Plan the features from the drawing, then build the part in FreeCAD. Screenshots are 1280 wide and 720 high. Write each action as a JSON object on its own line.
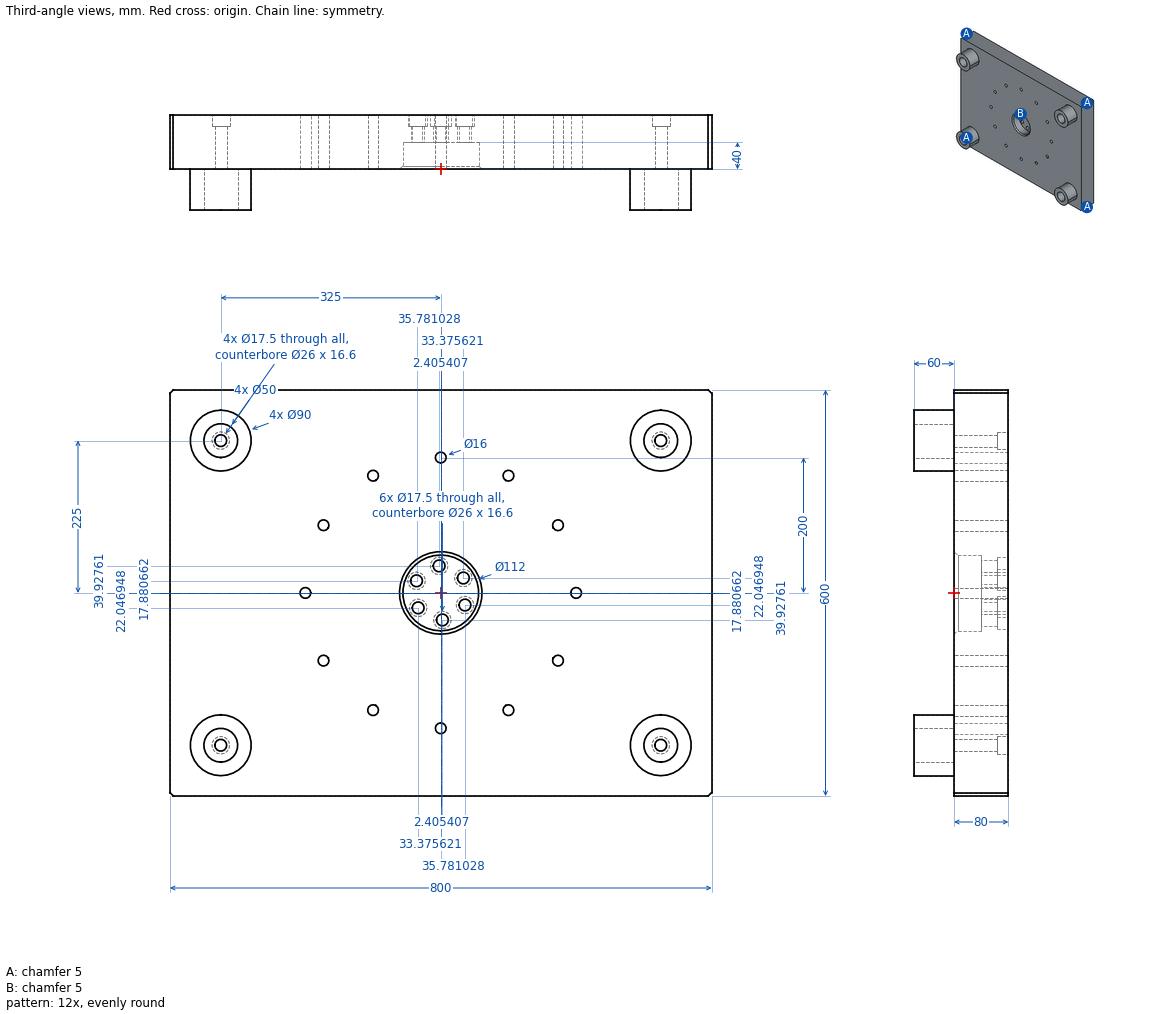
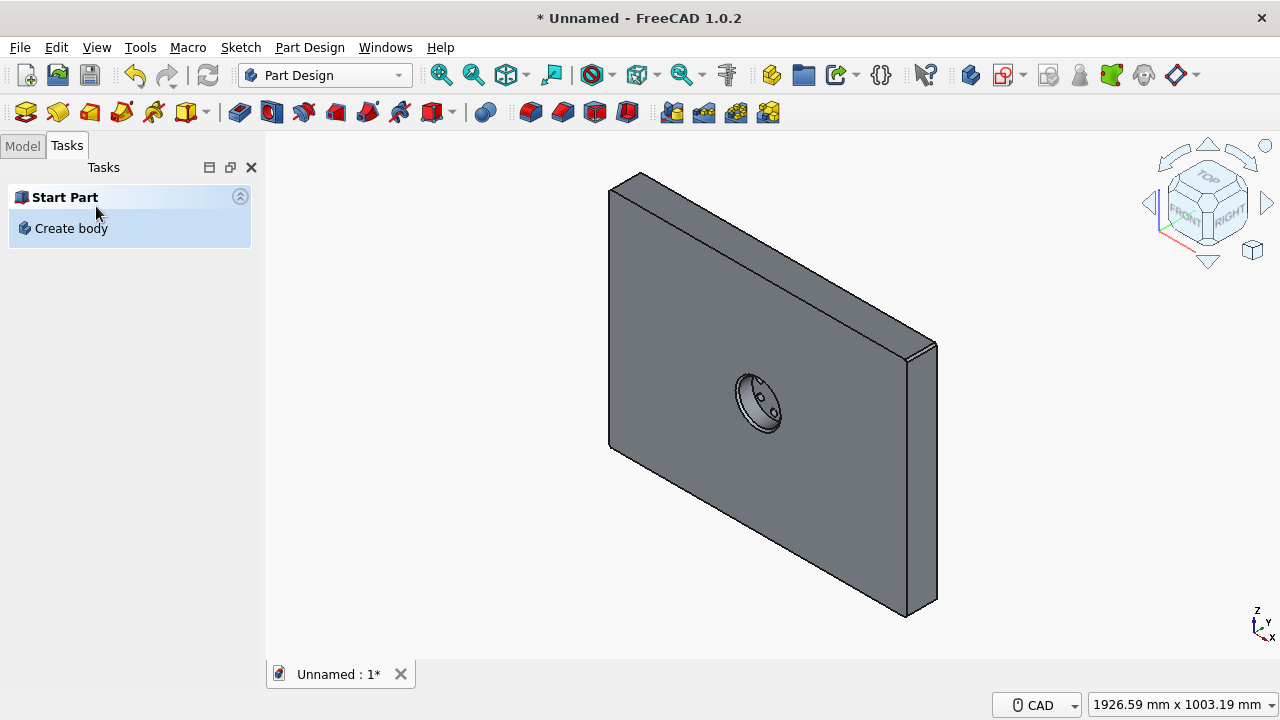
{"action": "left_click", "coordinate": [843, 415]}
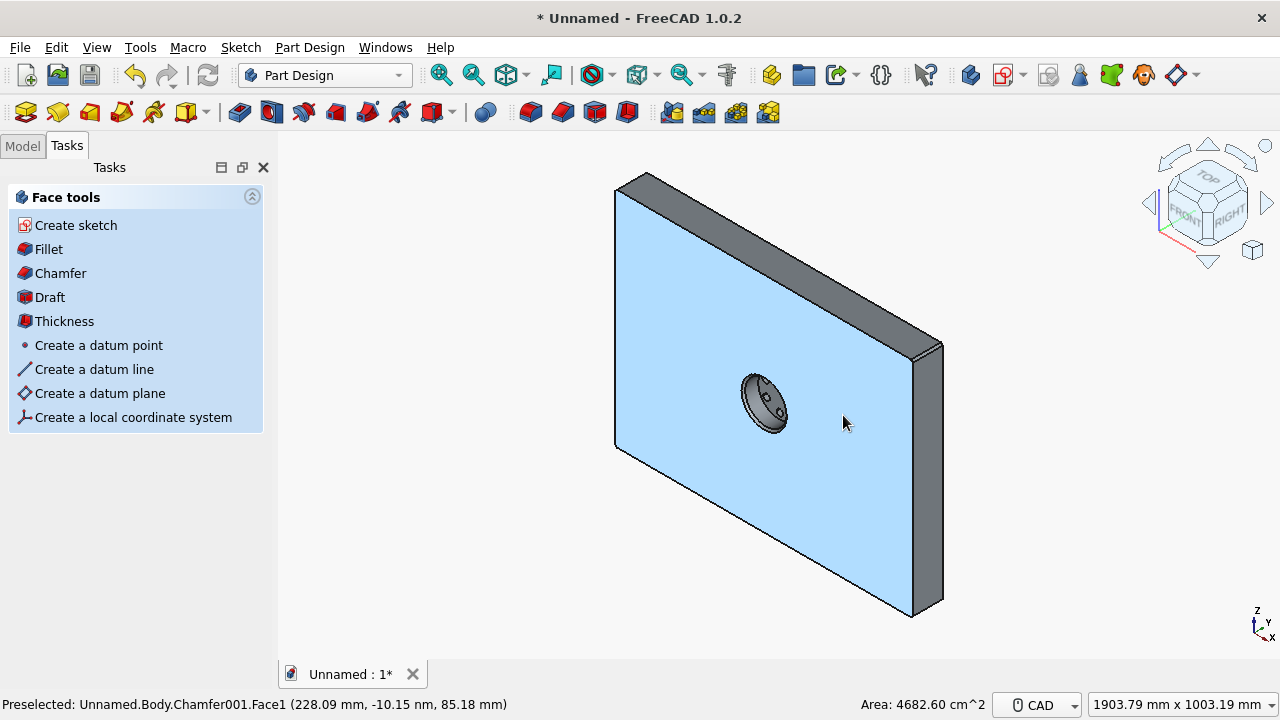
{"action": "left_click", "coordinate": [1004, 76]}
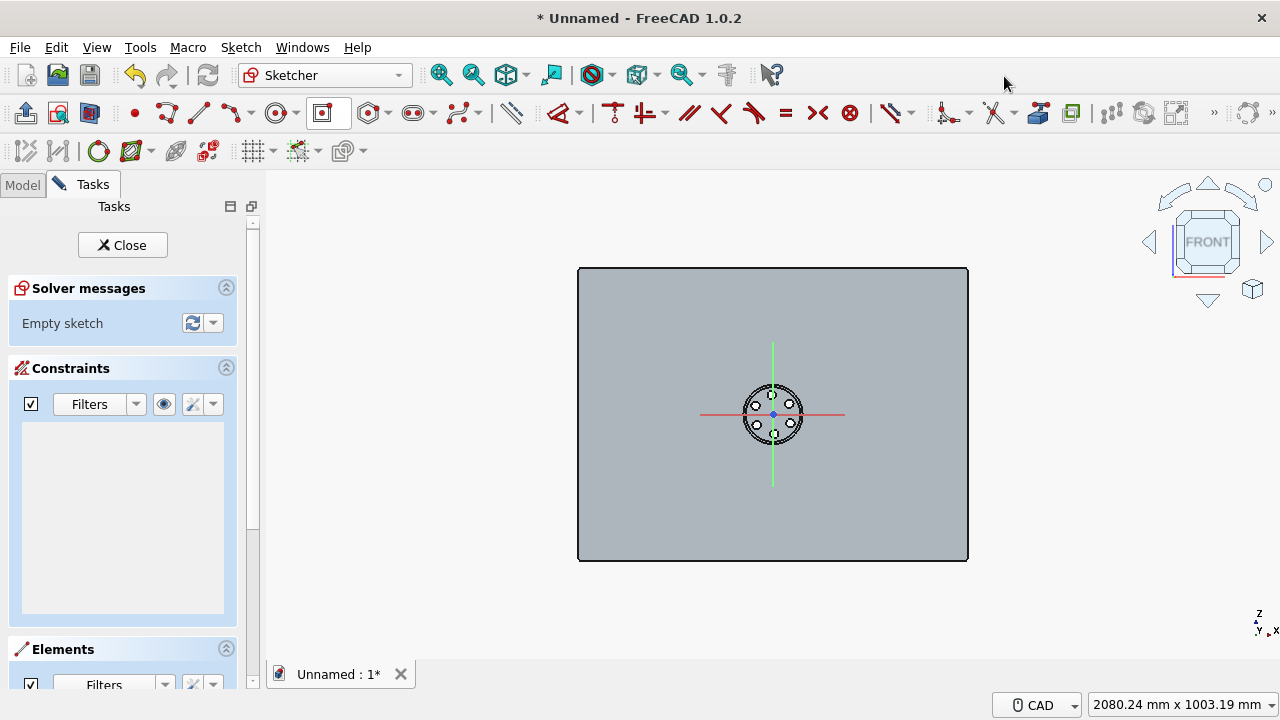
{"action": "key", "text": "g c"}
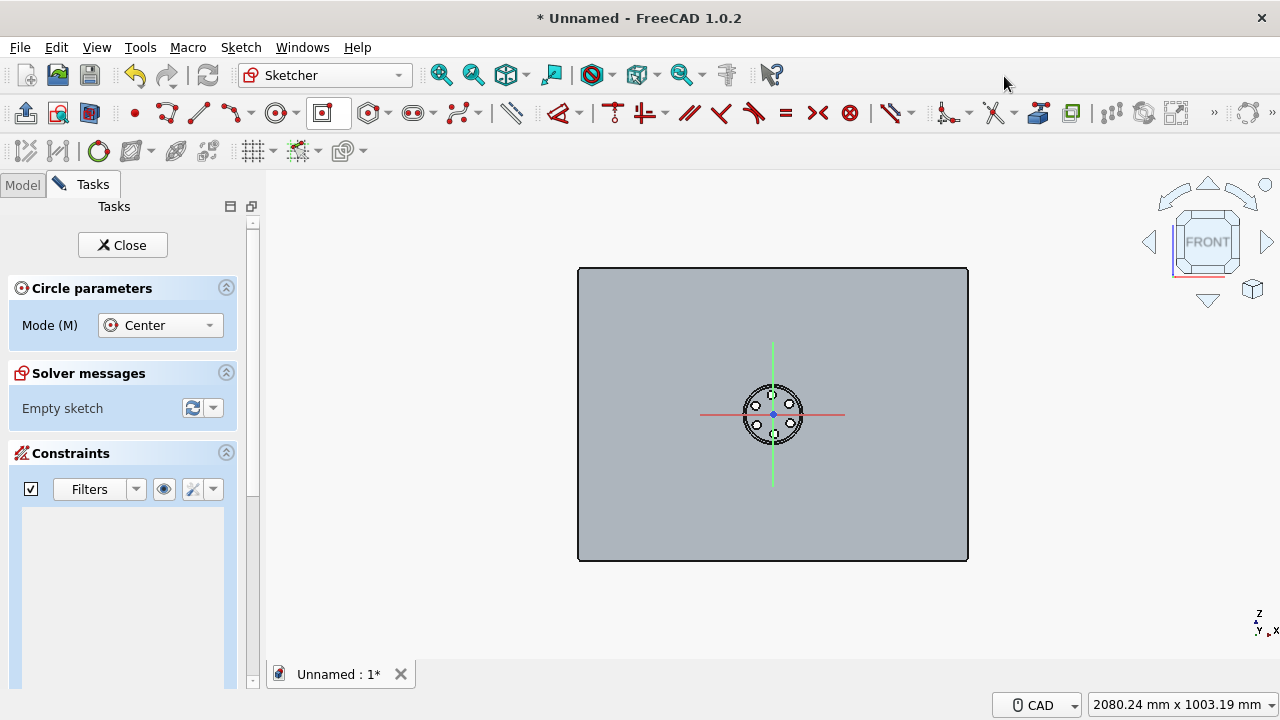
{"action": "left_click", "coordinate": [615, 305]}
{"action": "mouse_move", "coordinate": [630, 289]}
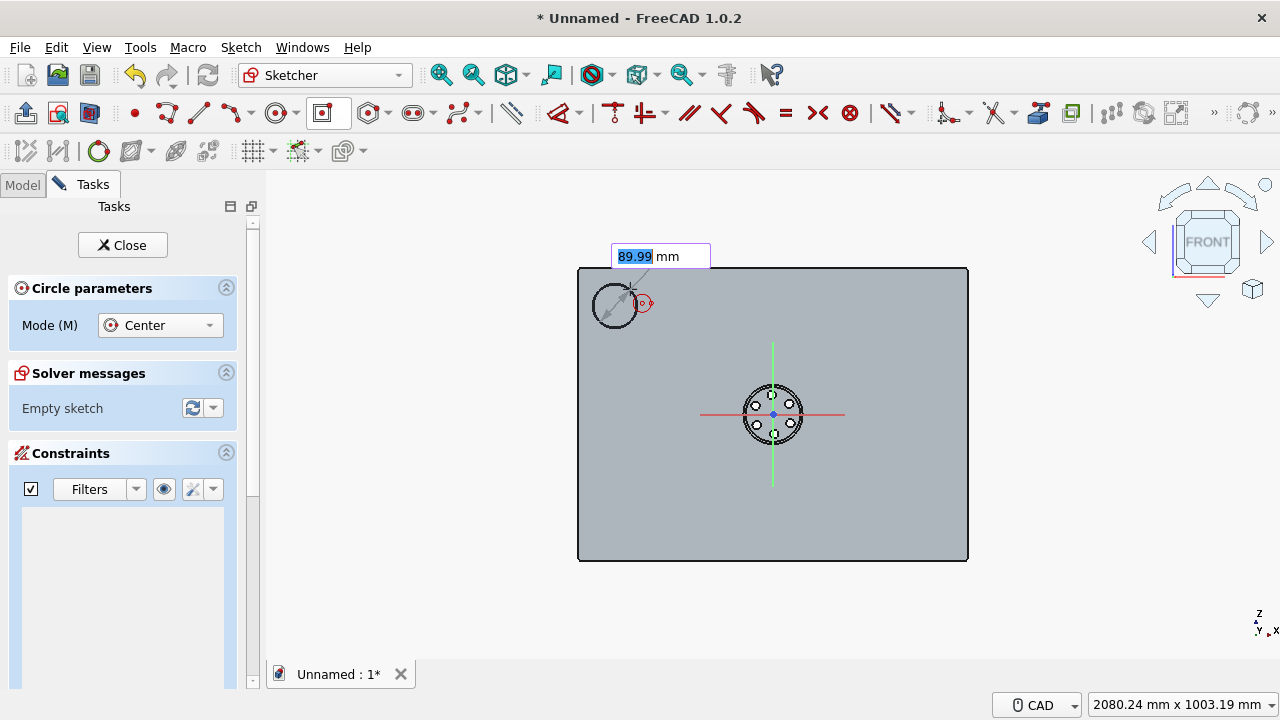
{"action": "type", "text": "90"}
{"action": "key", "text": "Return"}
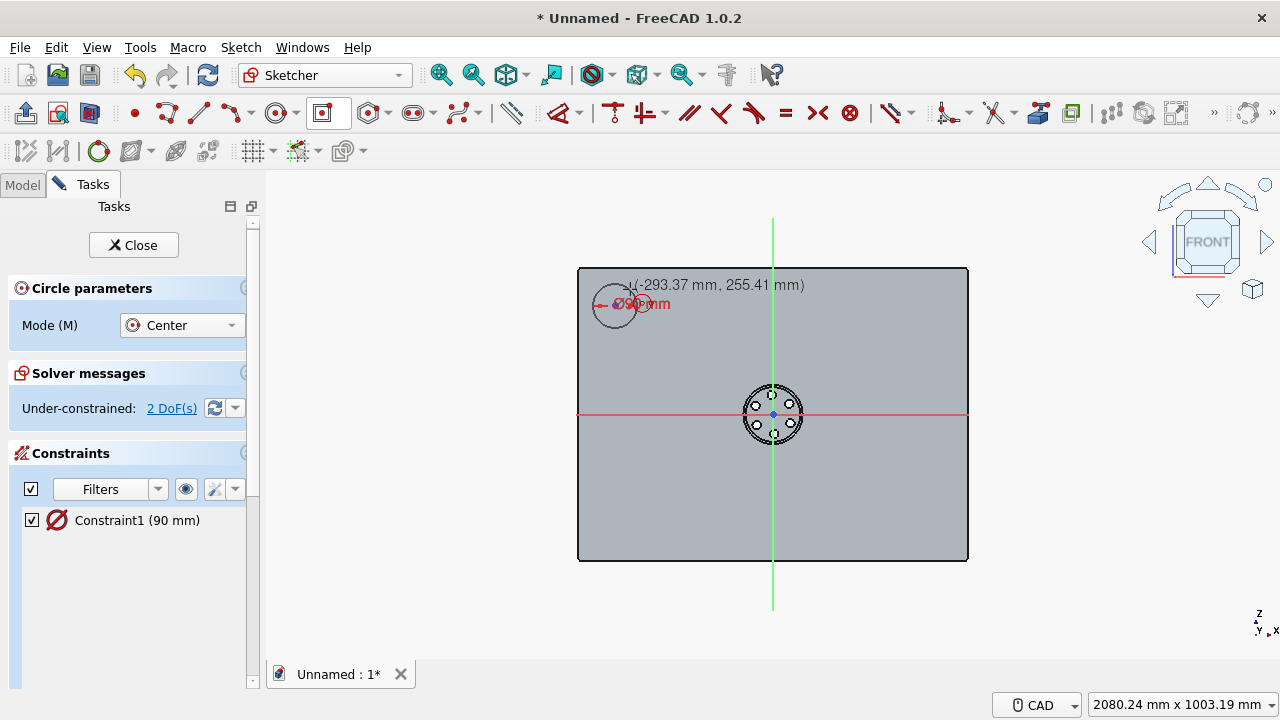
{"action": "left_click", "coordinate": [931, 305]}
{"action": "mouse_move", "coordinate": [947, 289]}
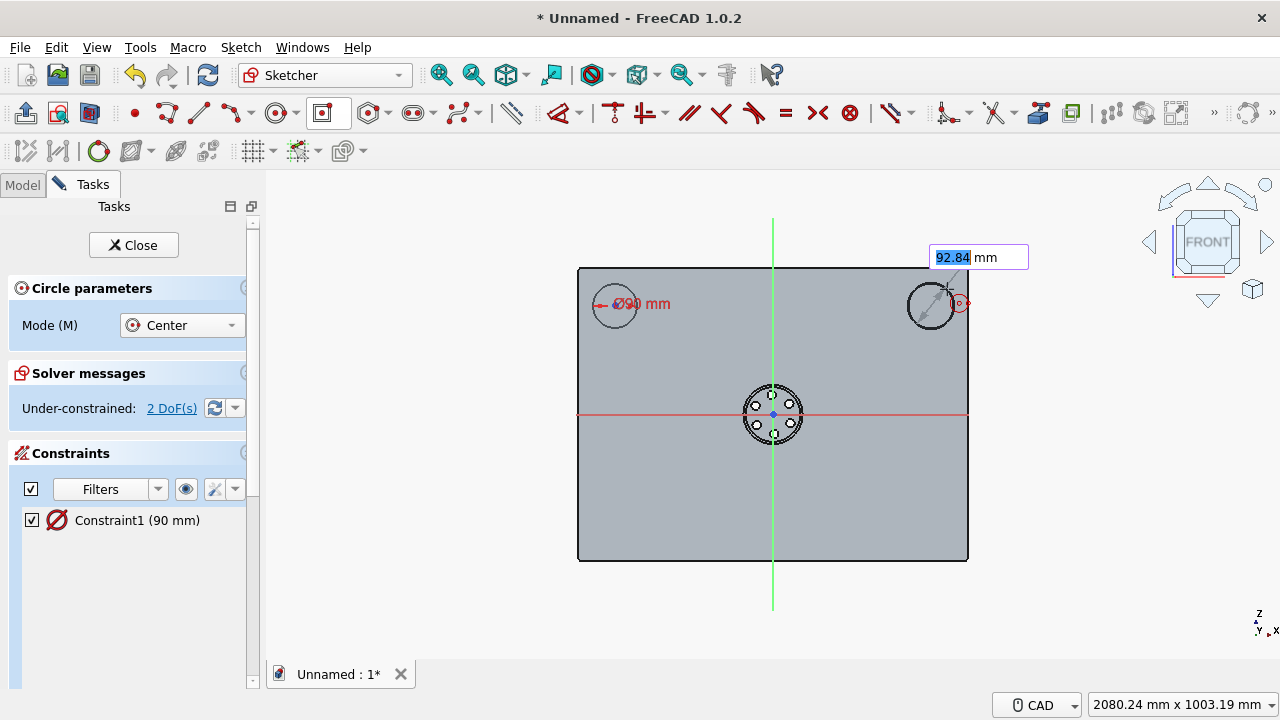
{"action": "type", "text": "90"}
{"action": "key", "text": "Return"}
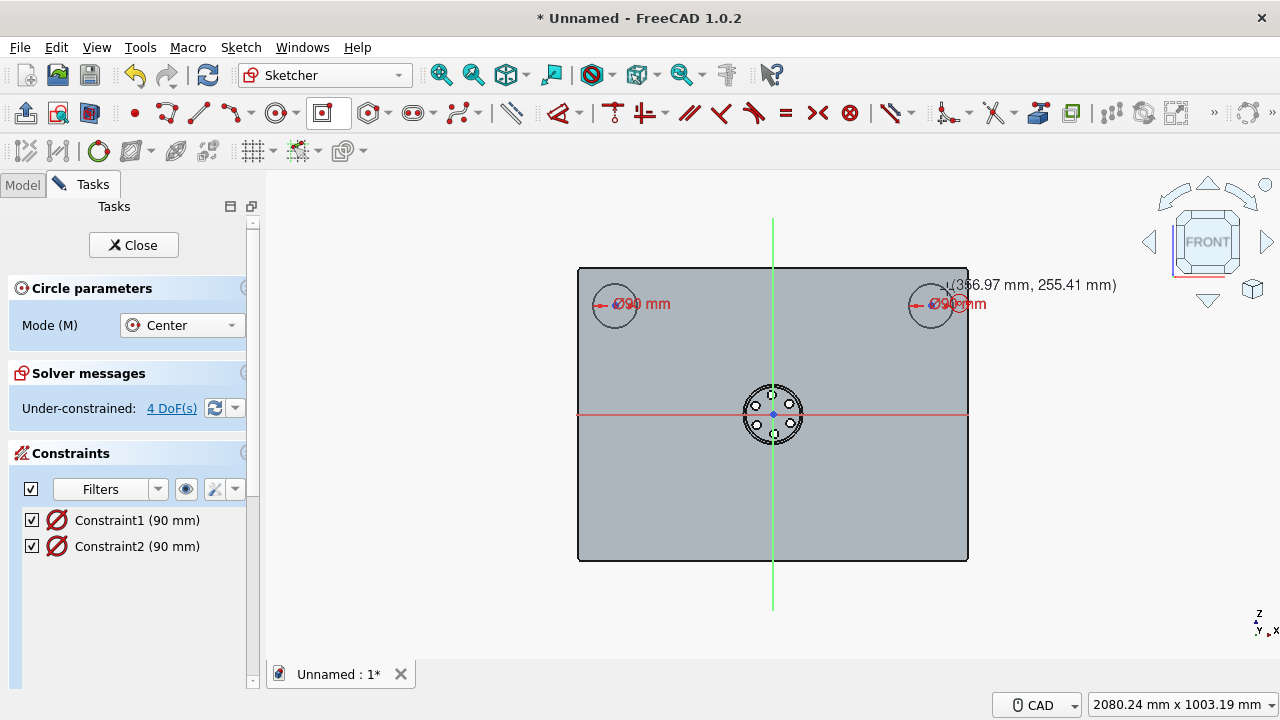
{"action": "left_click", "coordinate": [615, 524]}
{"action": "mouse_move", "coordinate": [630, 509]}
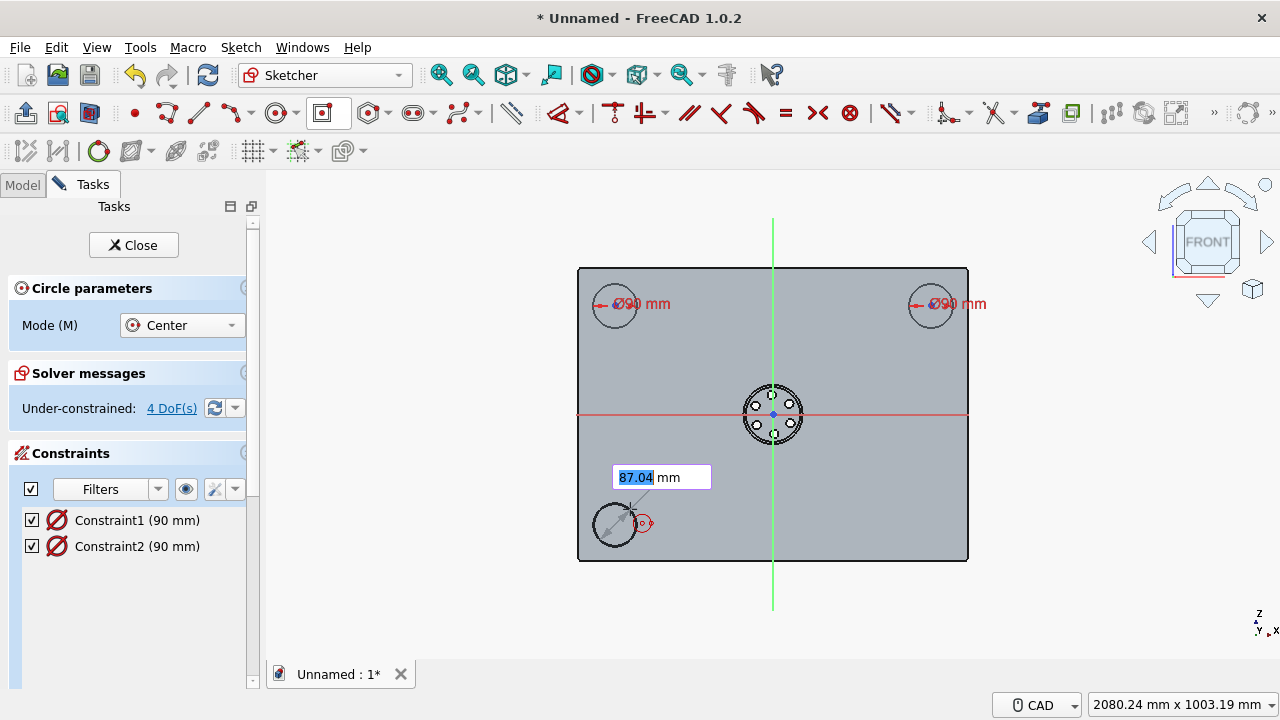
{"action": "type", "text": "90"}
{"action": "key", "text": "Return"}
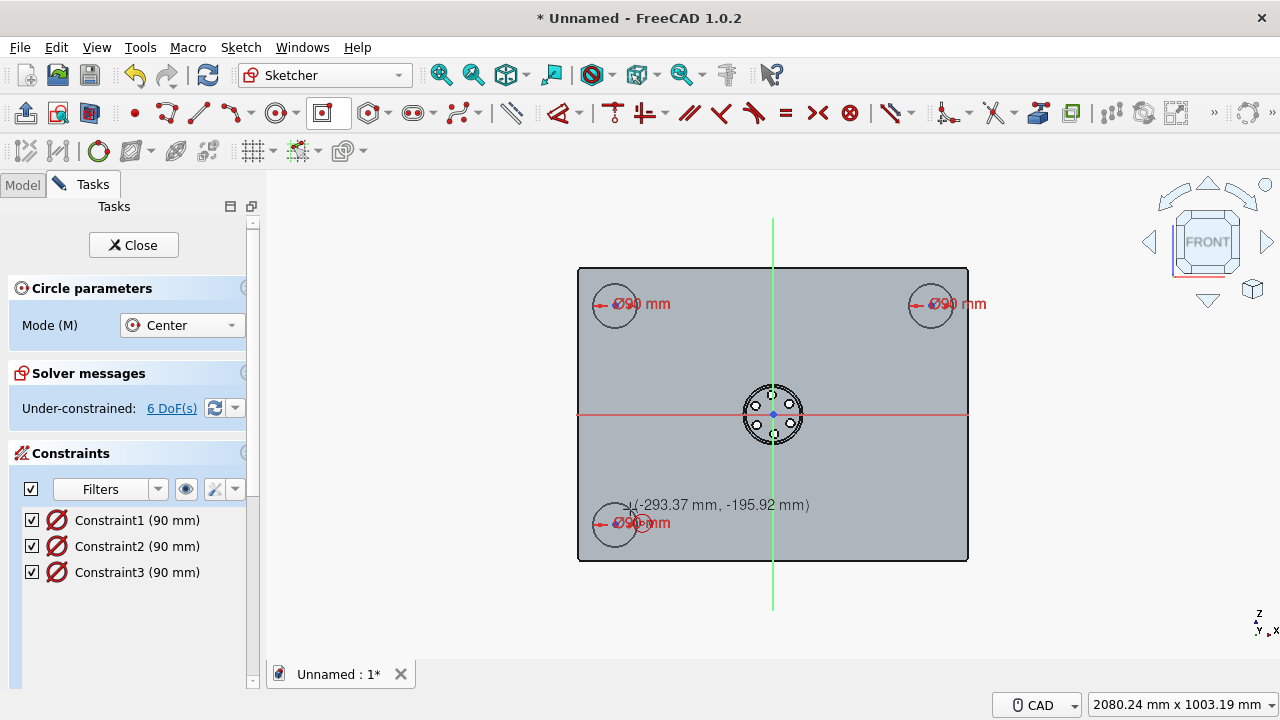
{"action": "left_click", "coordinate": [931, 524]}
{"action": "mouse_move", "coordinate": [947, 509]}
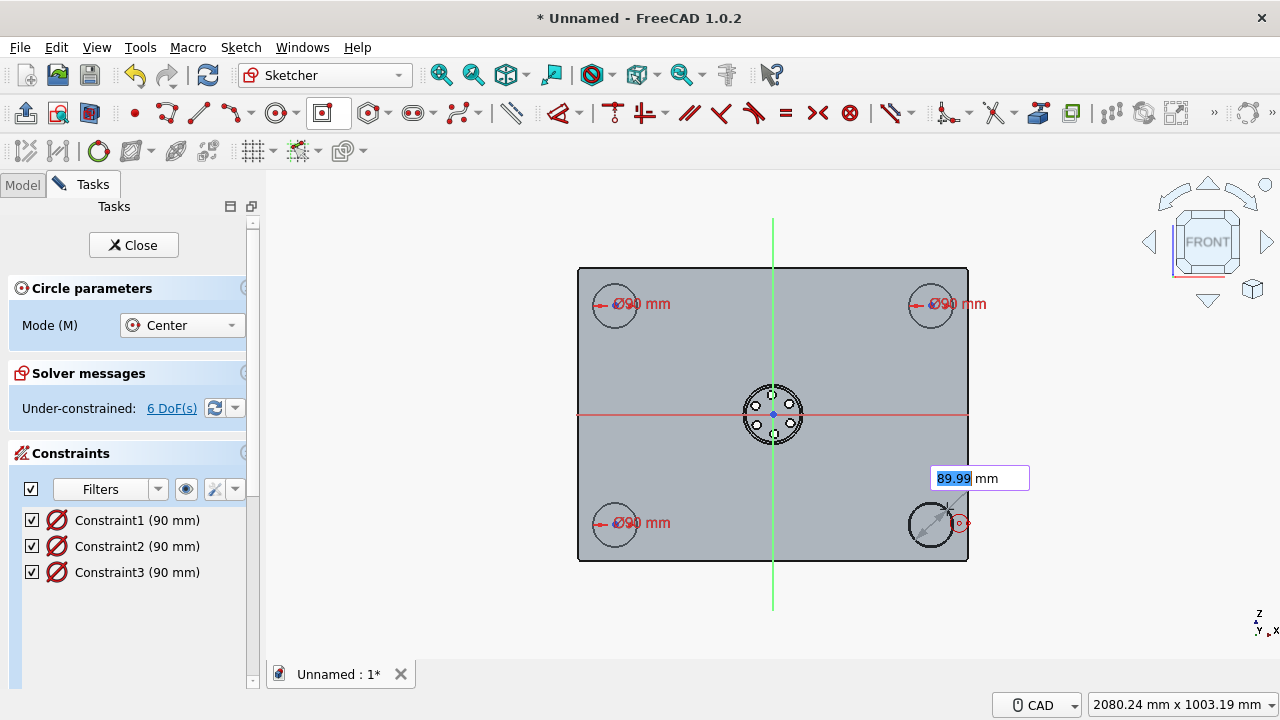
{"action": "type", "text": "90"}
{"action": "key", "text": "Return"}